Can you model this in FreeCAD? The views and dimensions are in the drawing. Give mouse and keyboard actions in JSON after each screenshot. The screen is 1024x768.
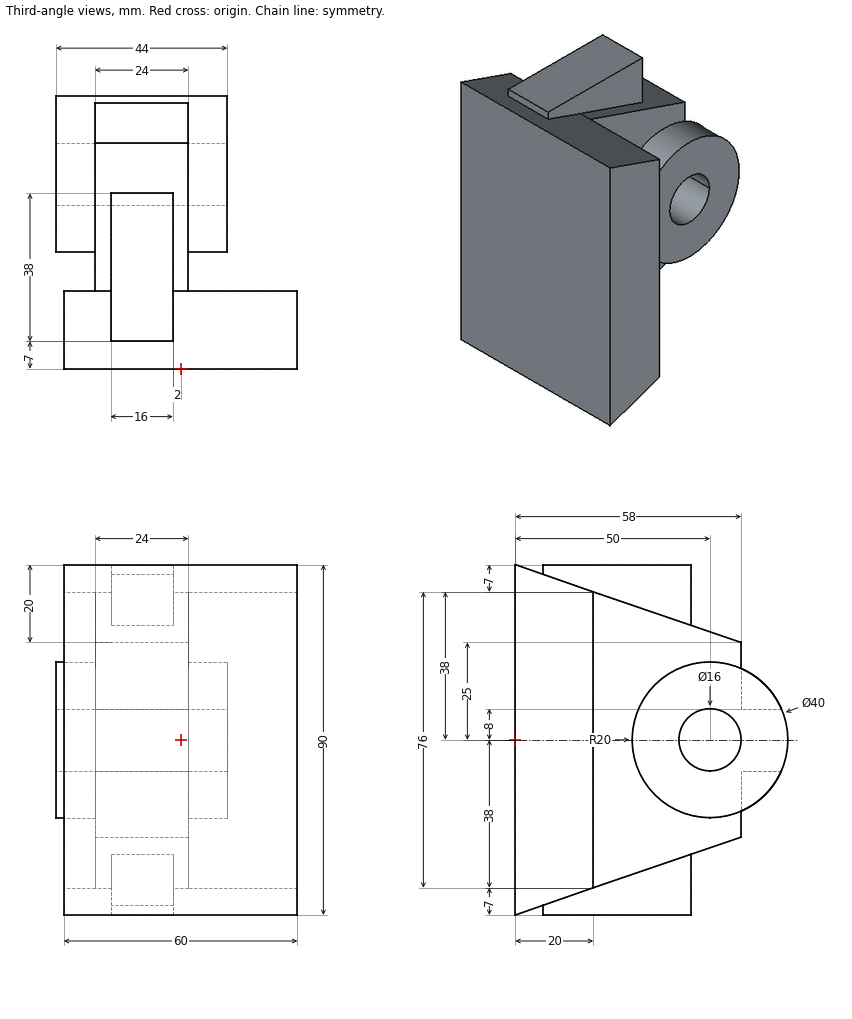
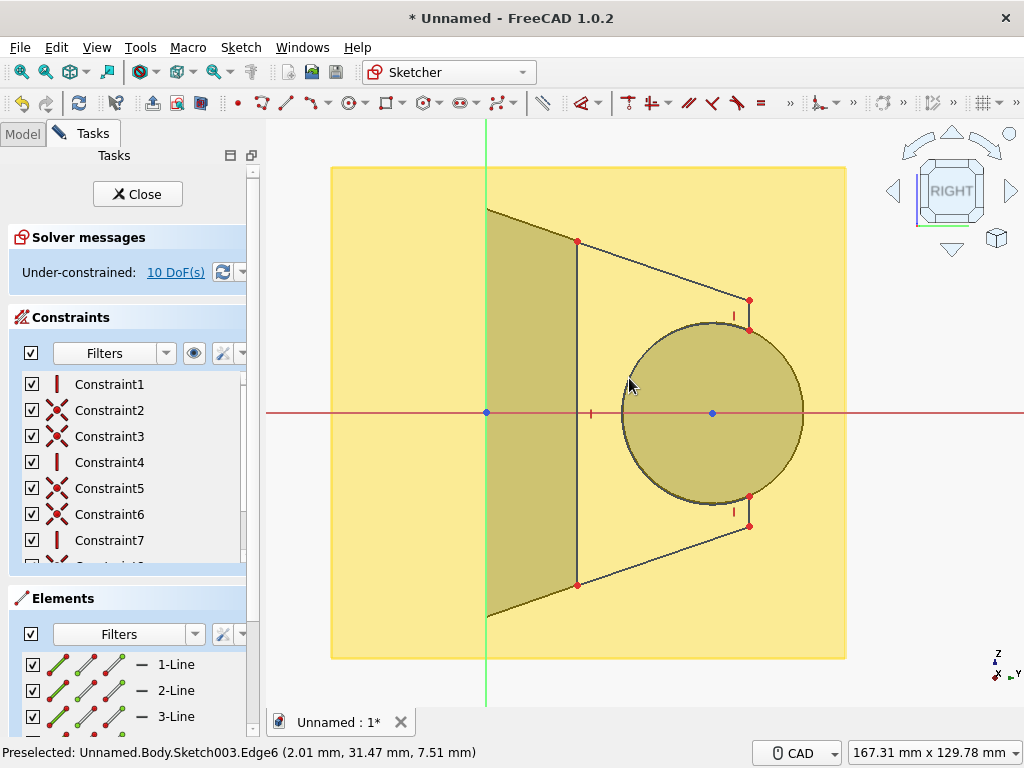
{"action": "left_click", "coordinate": [713, 414]}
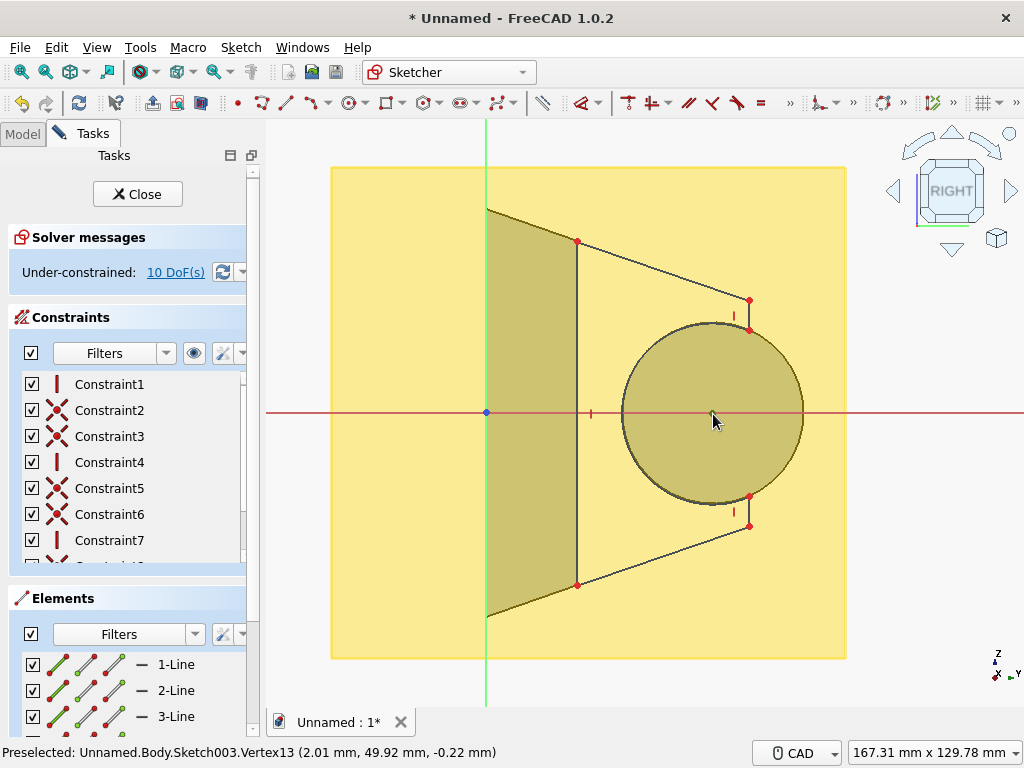
{"action": "left_click", "coordinate": [334, 413]}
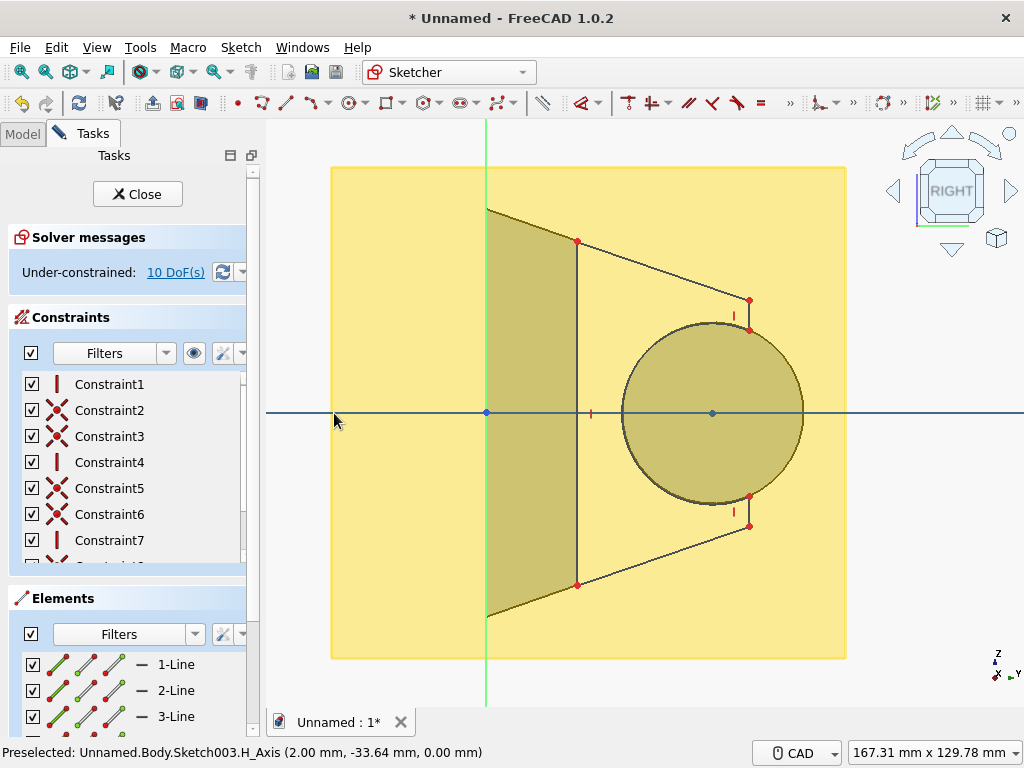
{"action": "left_click", "coordinate": [628, 104]}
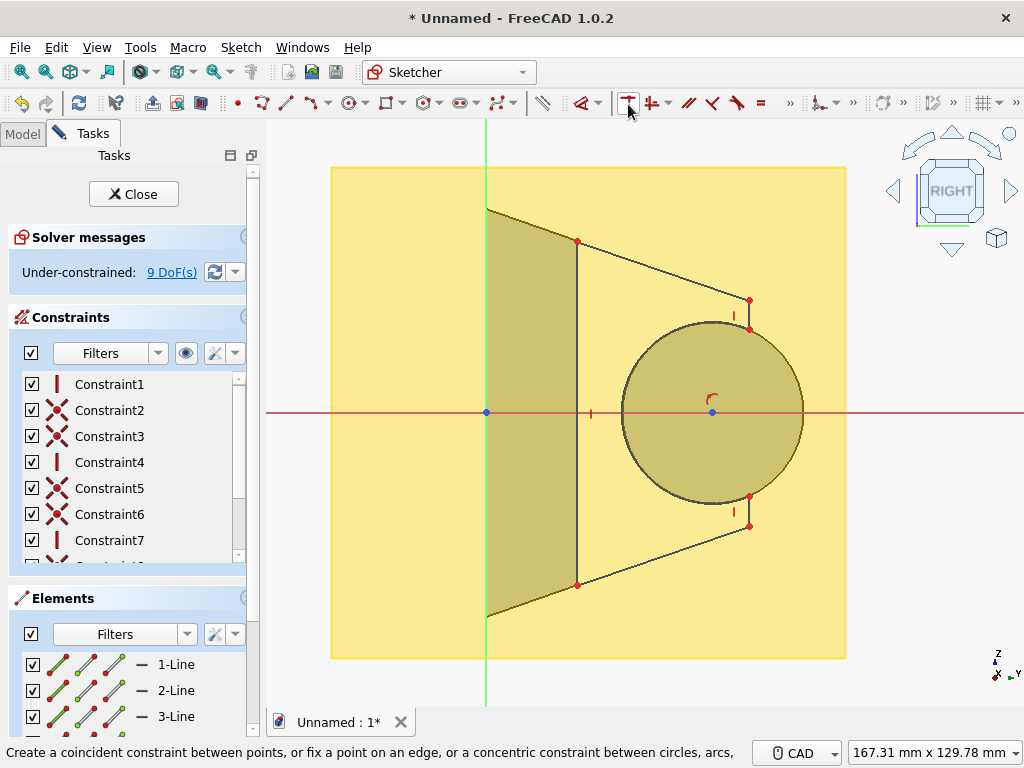
{"action": "left_click", "coordinate": [749, 301]}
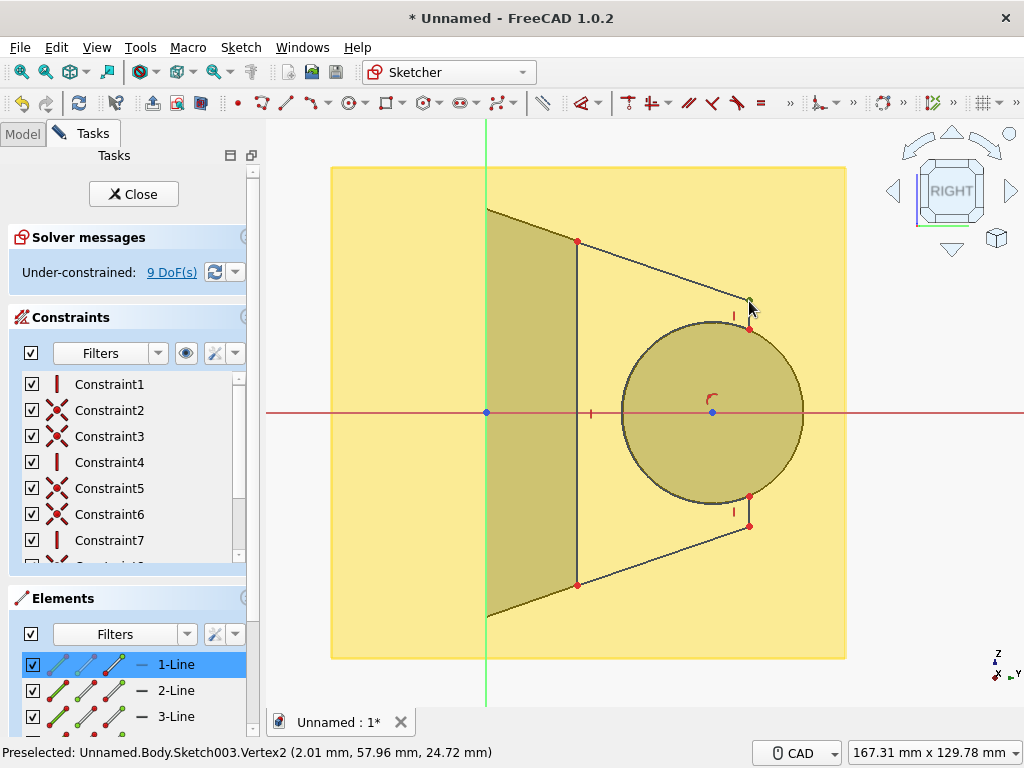
{"action": "left_click", "coordinate": [749, 527]}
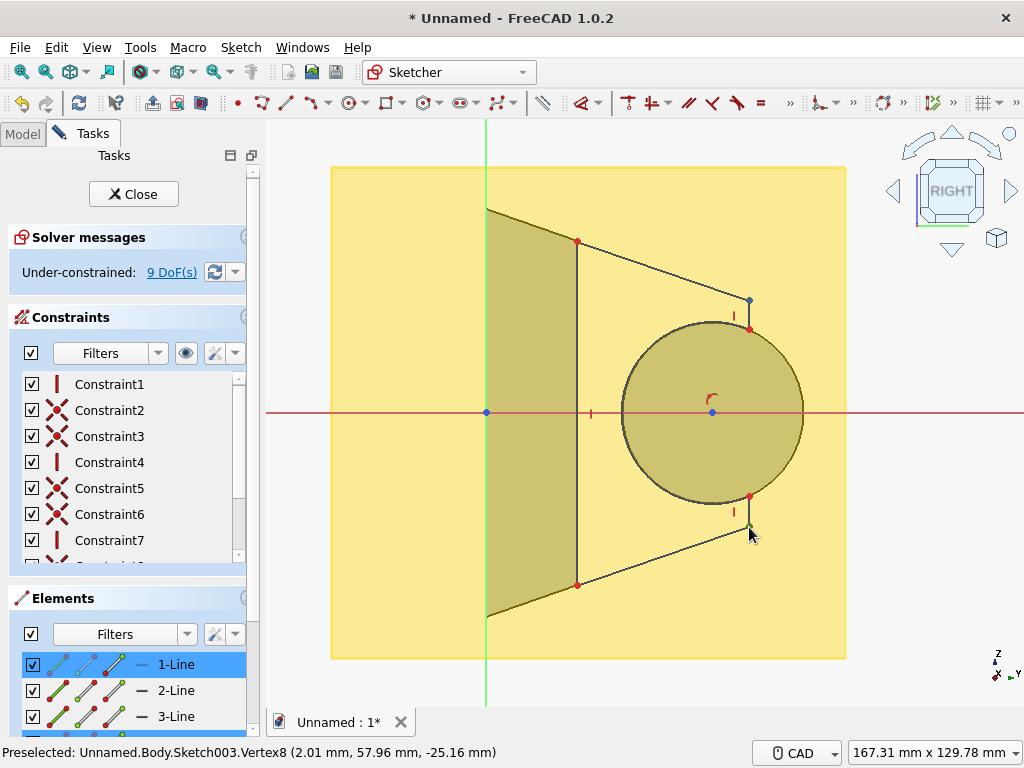
{"action": "left_click", "coordinate": [334, 413]}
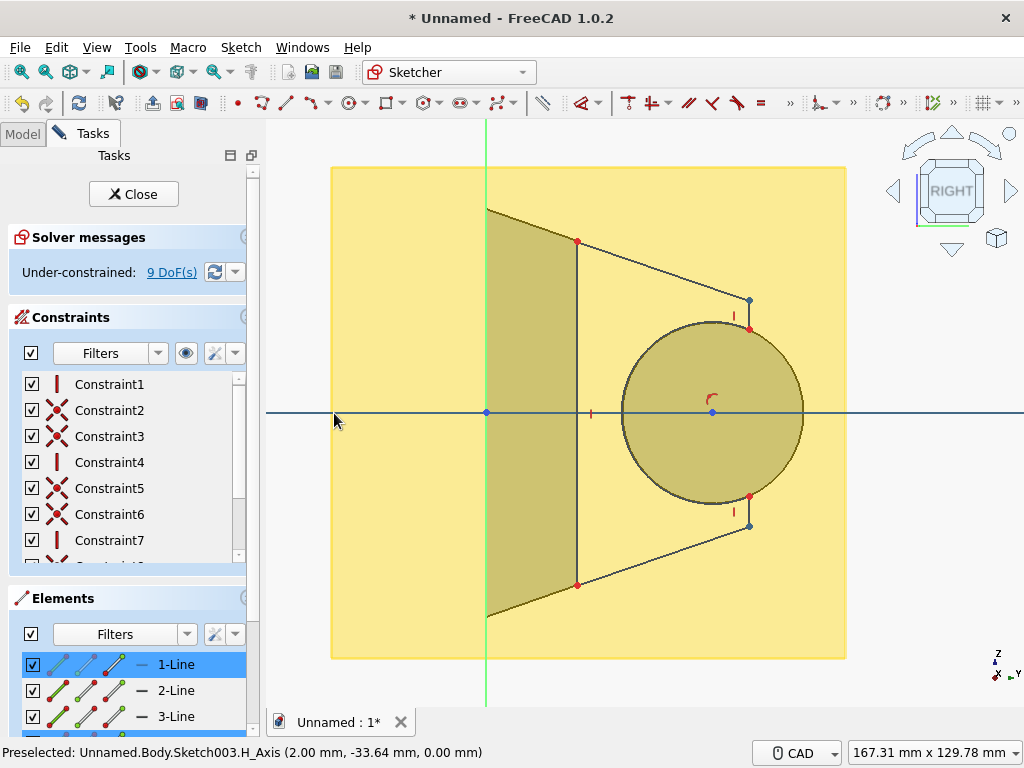
{"action": "key", "text": "s"}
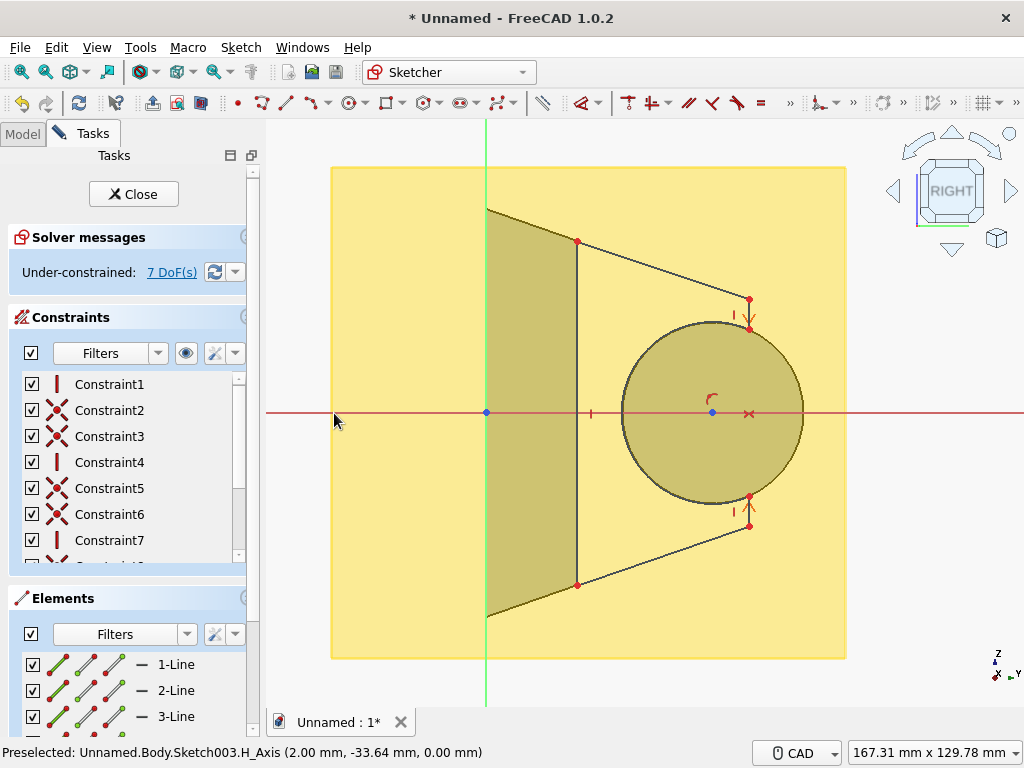
{"action": "key", "text": "d"}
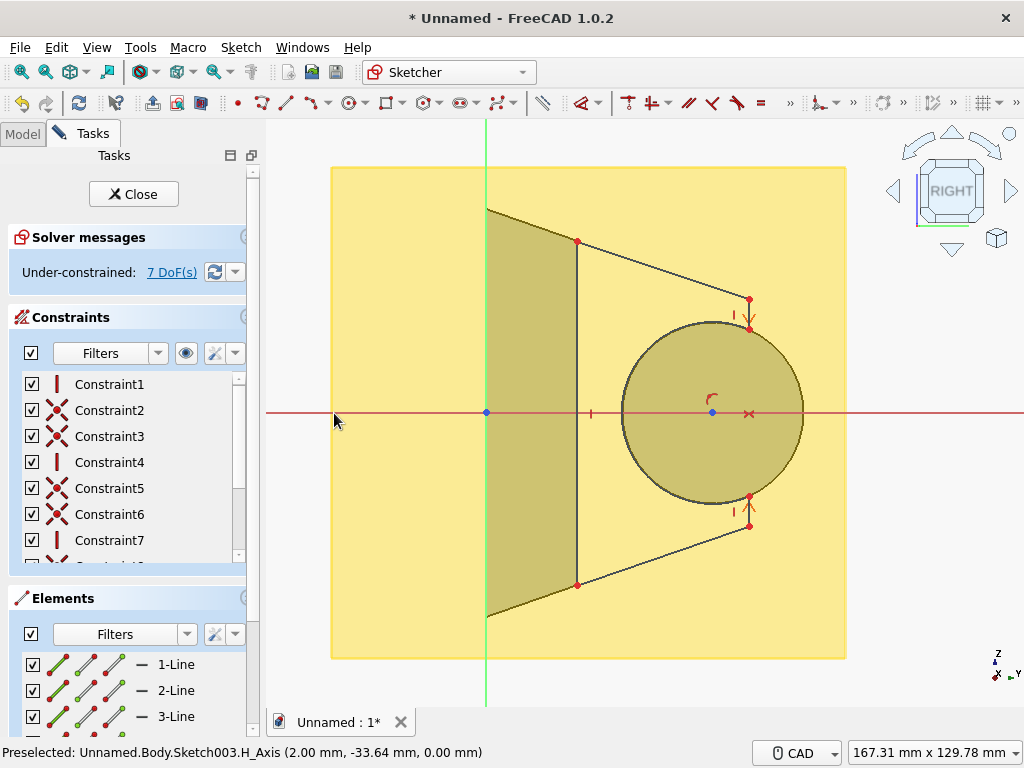
{"action": "left_click", "coordinate": [649, 348]}
{"action": "left_click", "coordinate": [627, 325]}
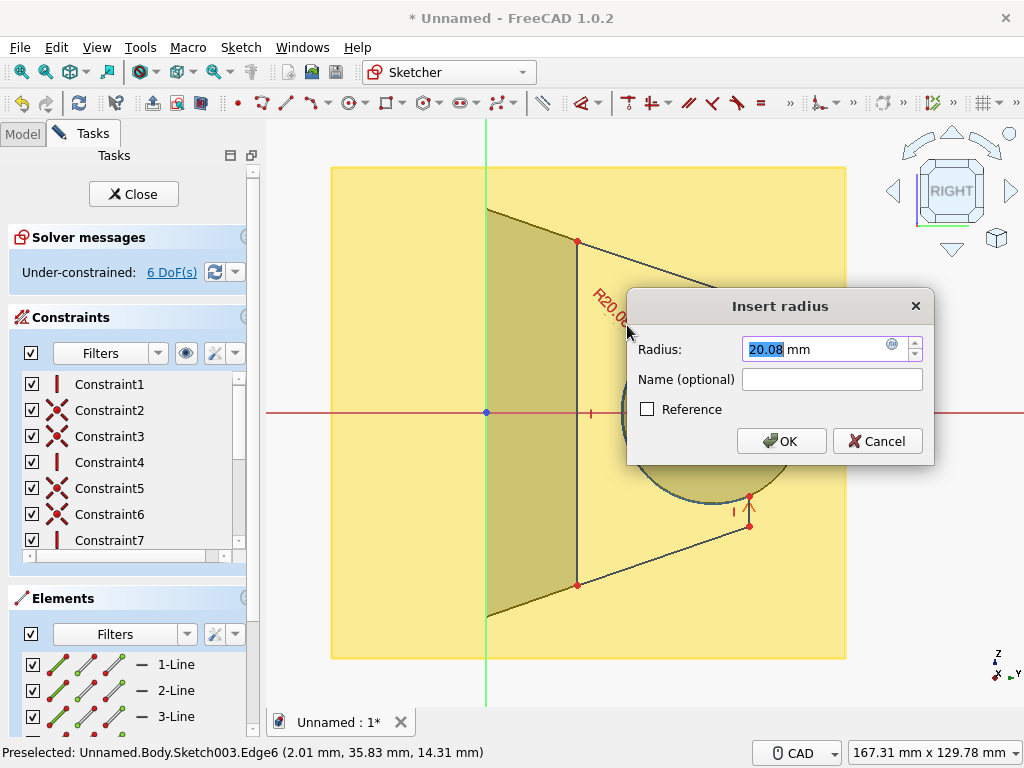
{"action": "type", "text": "20"}
{"action": "key", "text": "Return"}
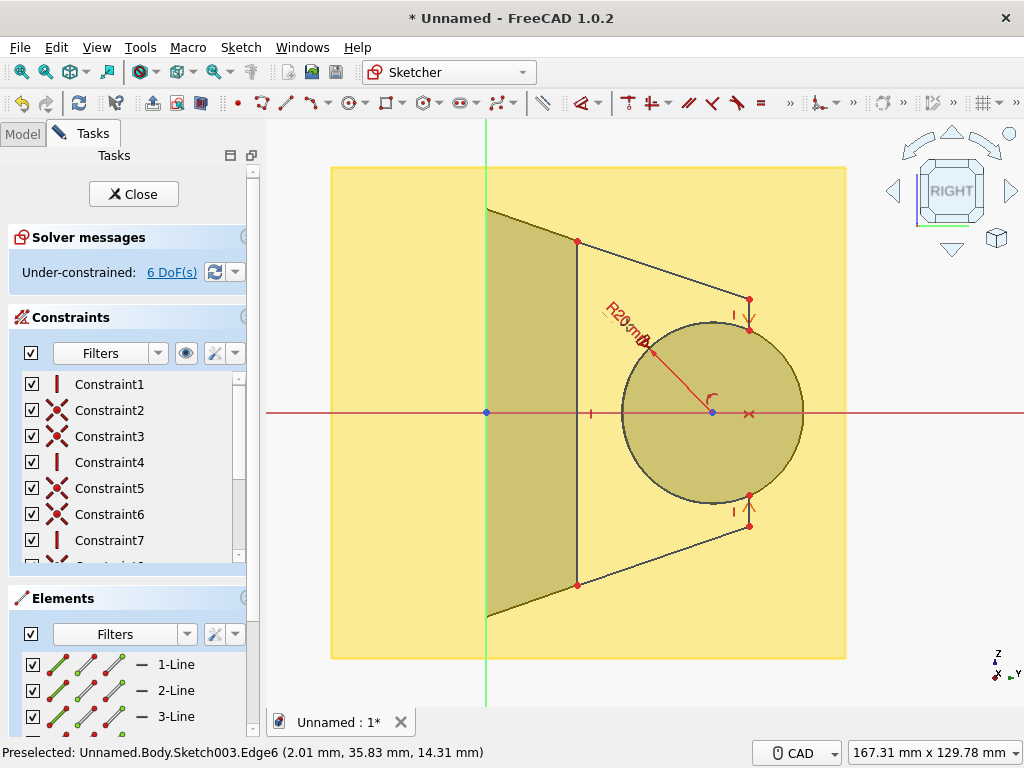
{"action": "left_click", "coordinate": [577, 345]}
{"action": "left_click", "coordinate": [543, 335]}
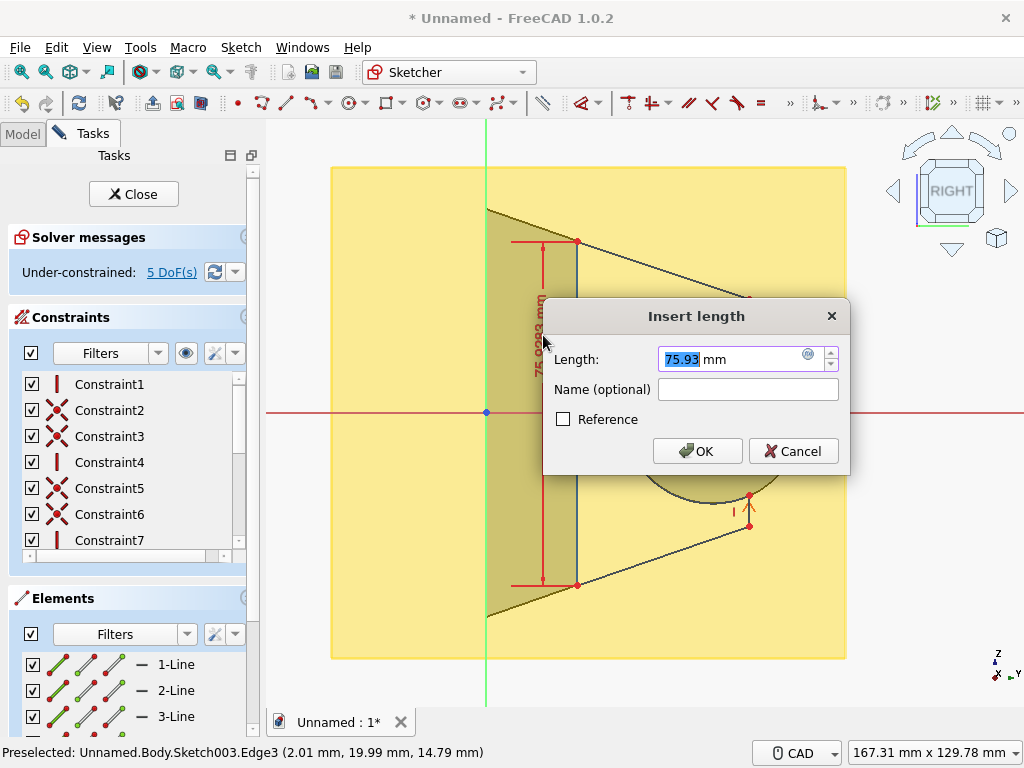
{"action": "type", "text": "76"}
{"action": "key", "text": "Return"}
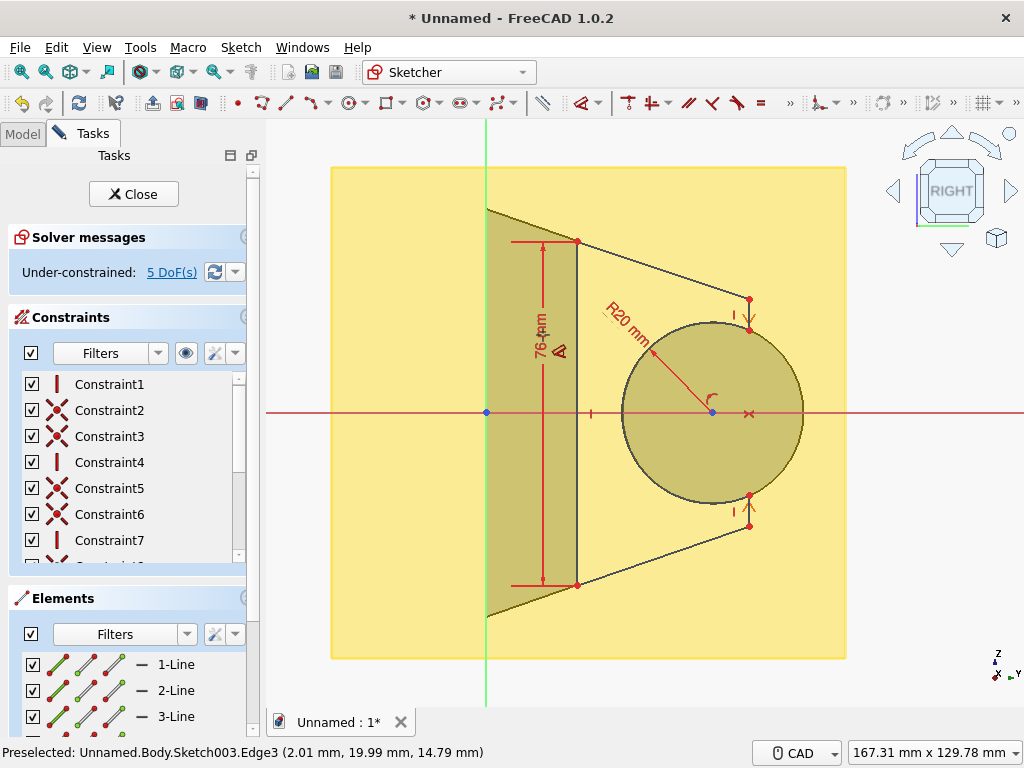
{"action": "left_click", "coordinate": [749, 330]}
{"action": "left_click", "coordinate": [618, 296]}